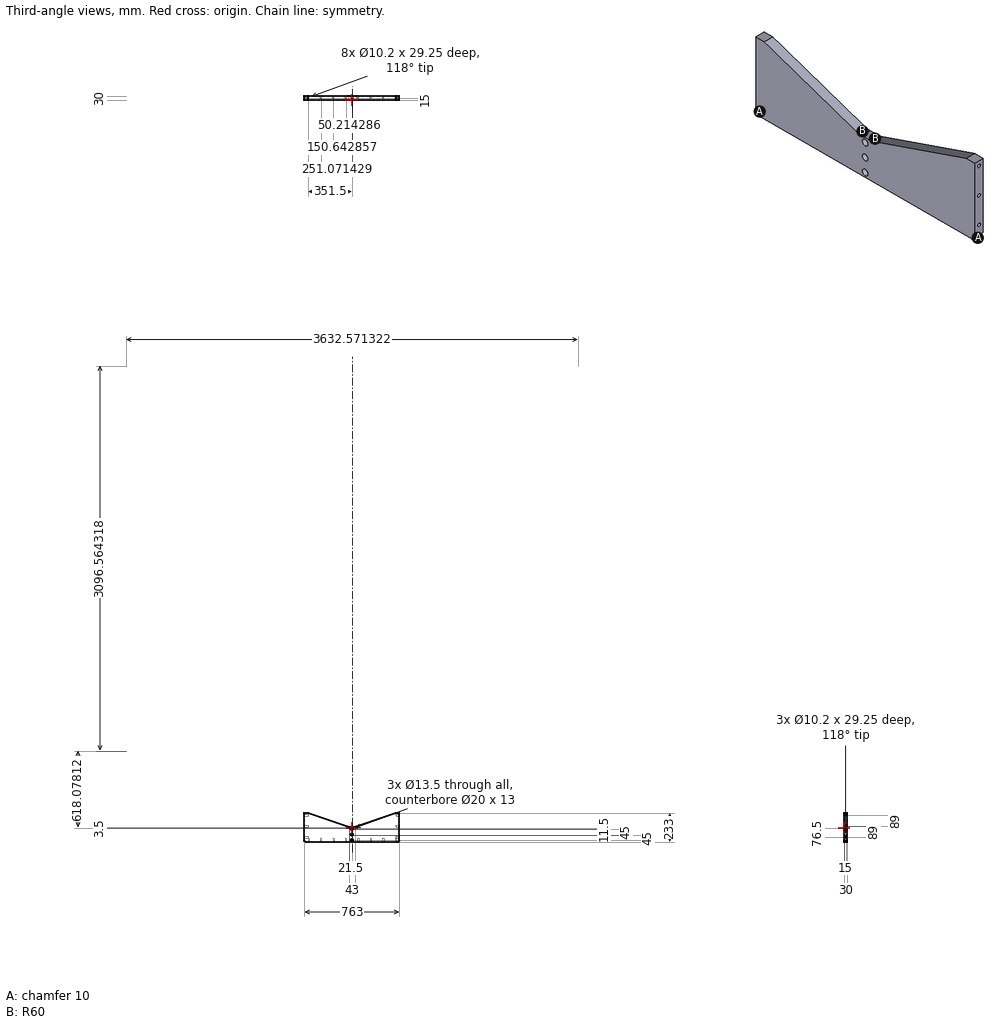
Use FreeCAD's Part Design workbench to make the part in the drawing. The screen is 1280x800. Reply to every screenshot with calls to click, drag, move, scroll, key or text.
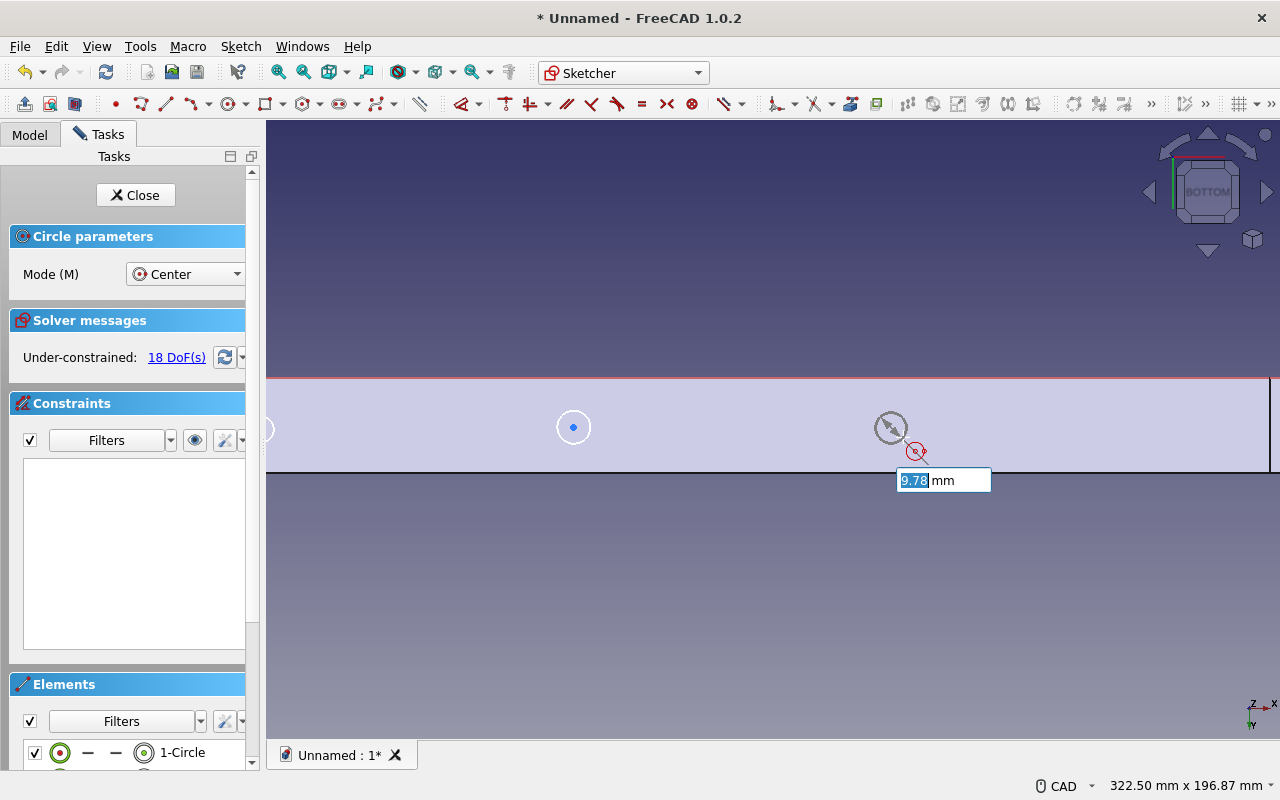
click(902, 437)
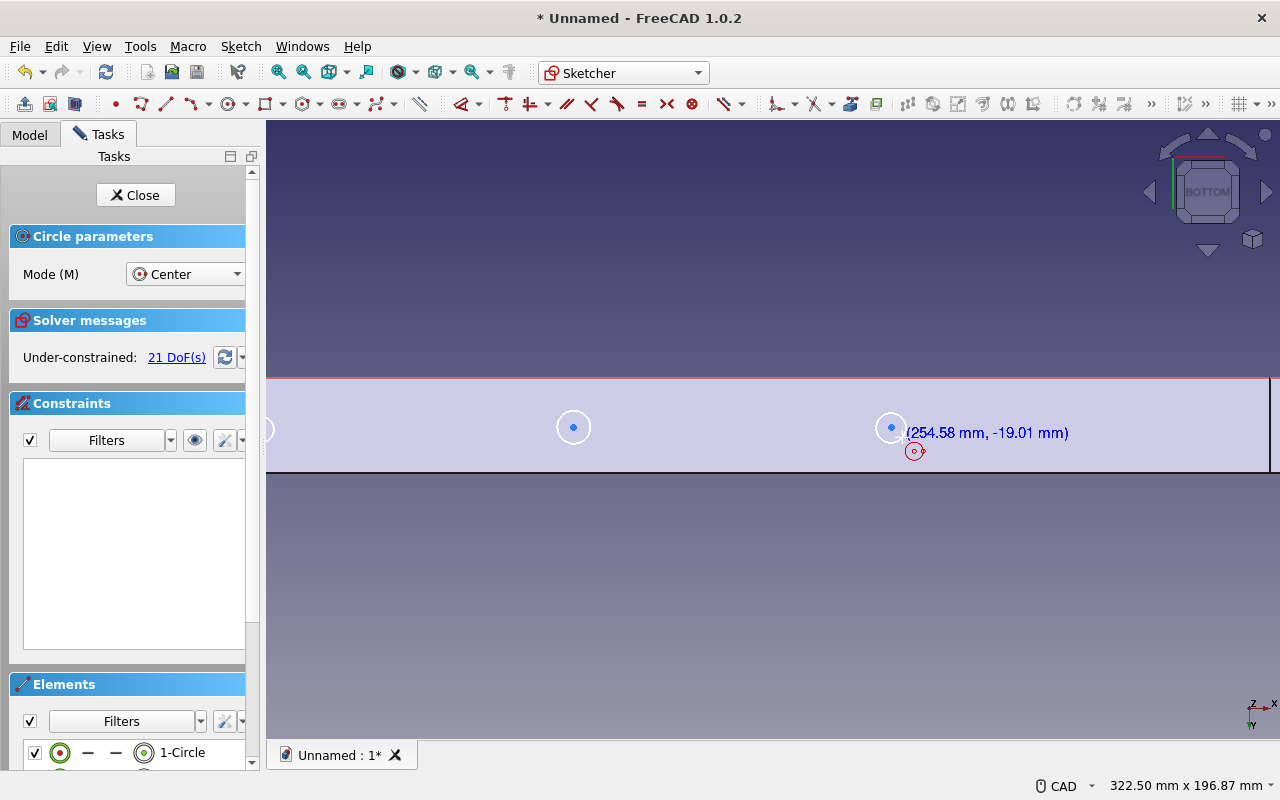
scroll(902, 436, down, 7)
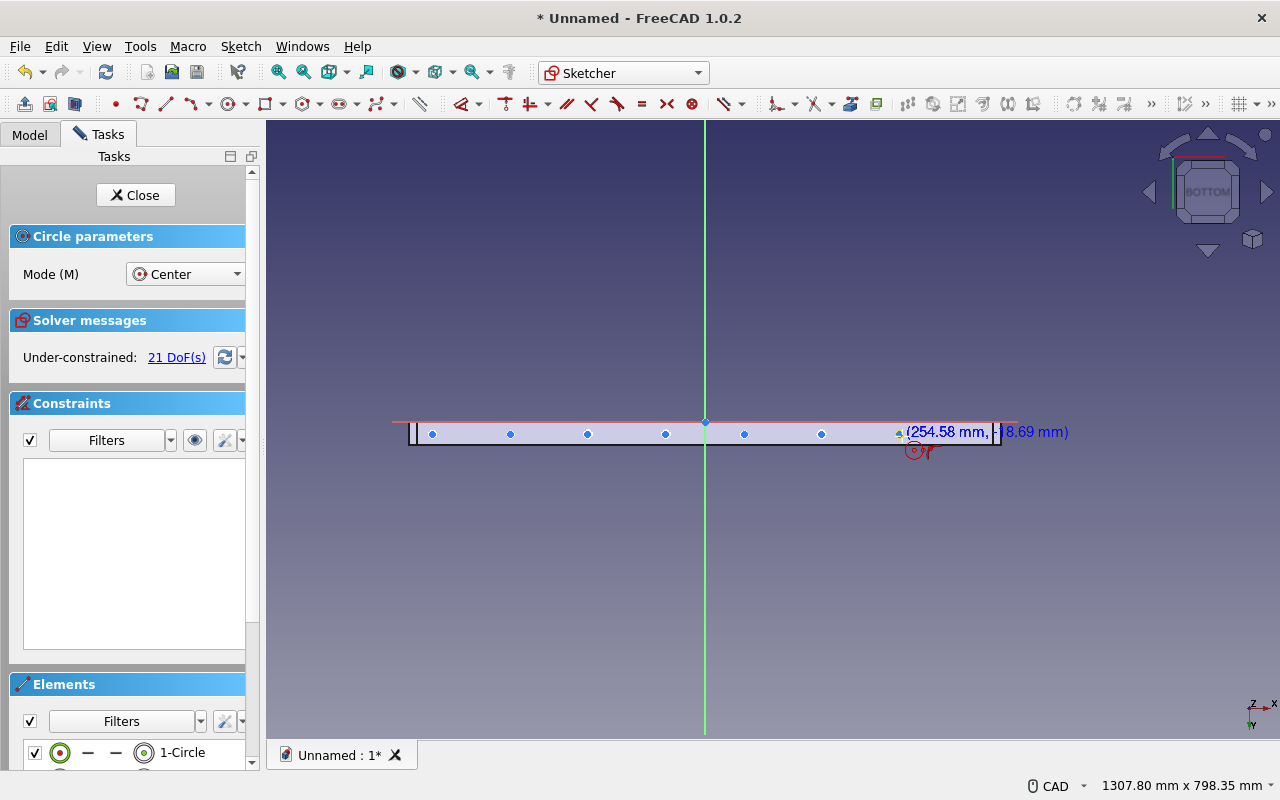
scroll(978, 434, up, 9)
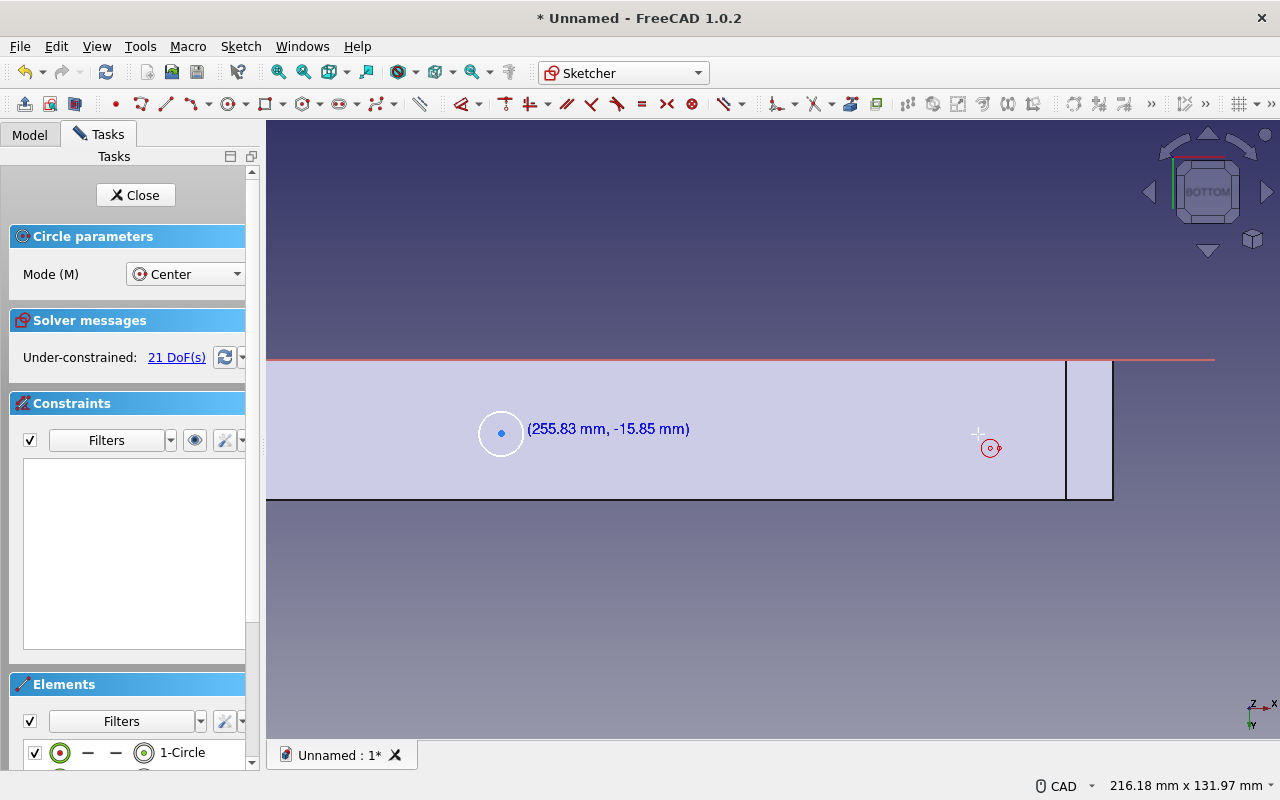
scroll(978, 434, down, 9)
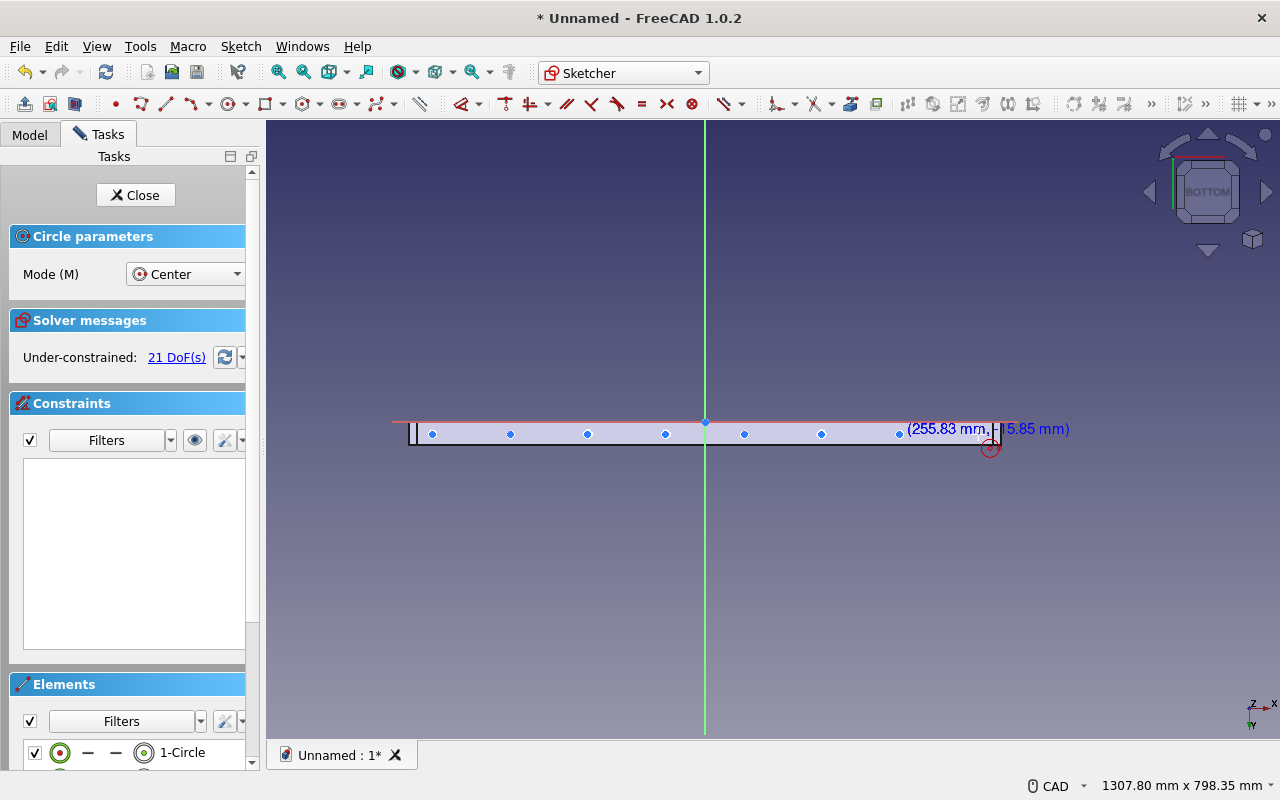
scroll(978, 434, up, 2)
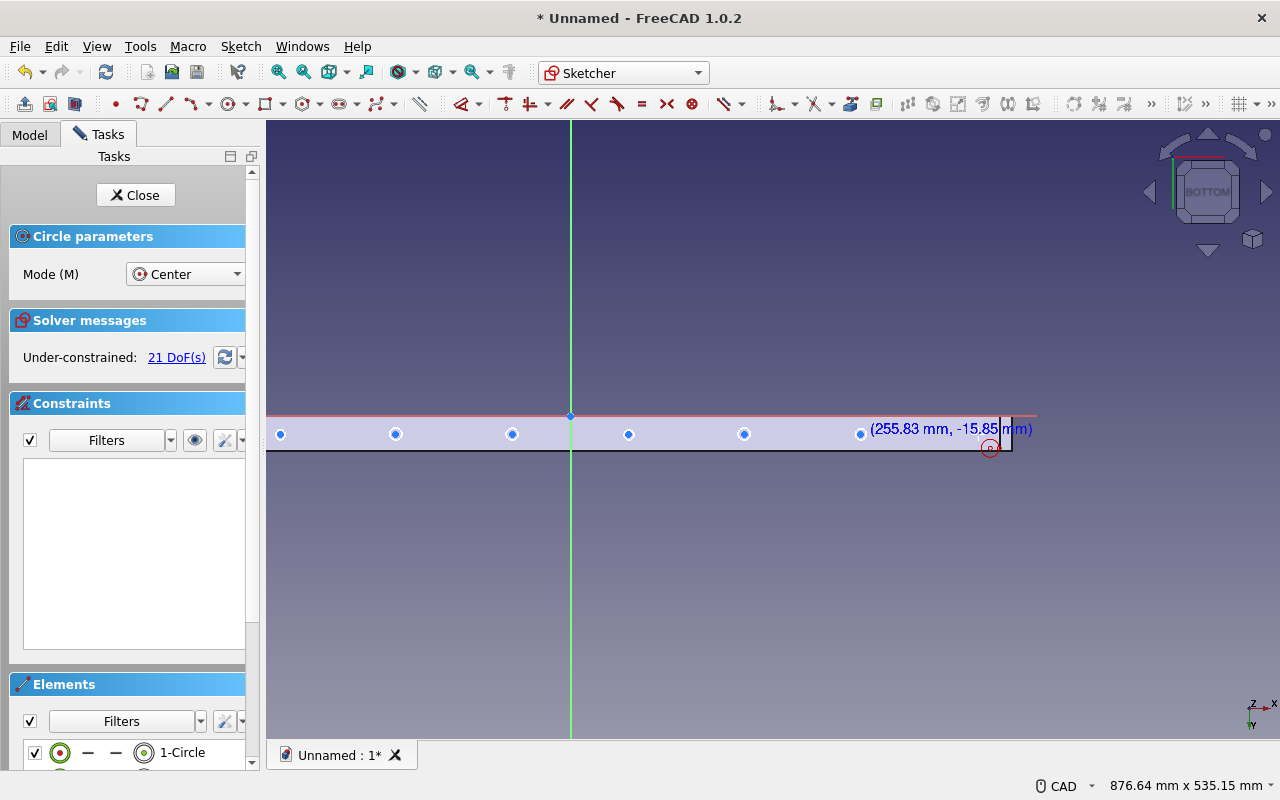
click(977, 433)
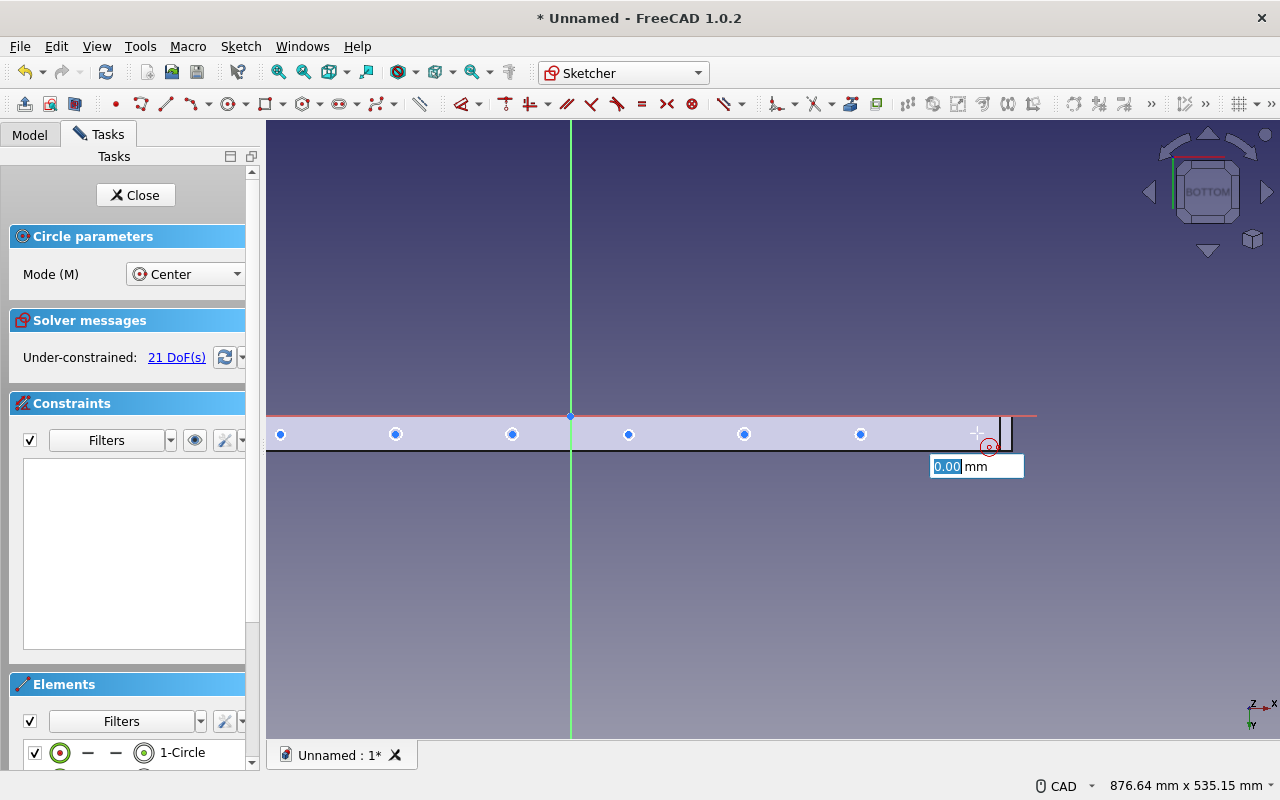
scroll(981, 438, up, 5)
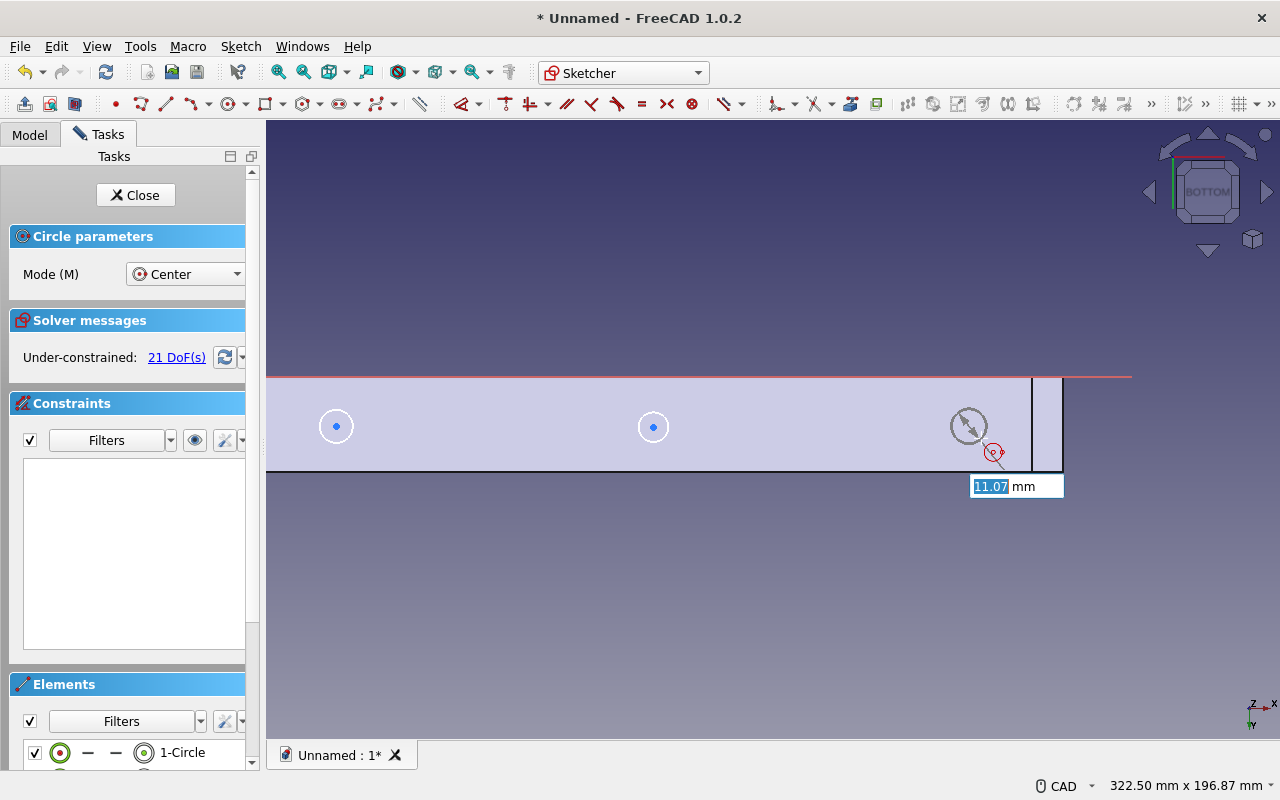
click(980, 436)
key(Escape)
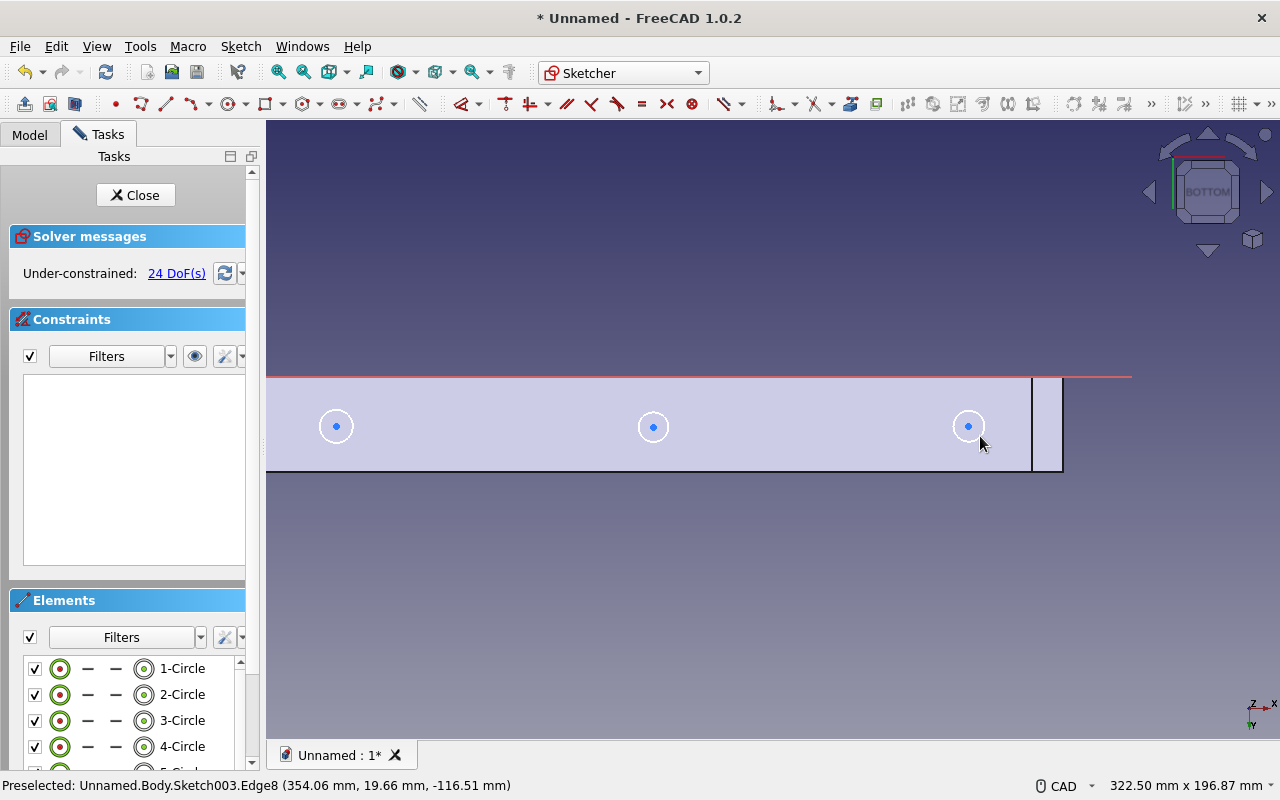
scroll(980, 436, down, 7)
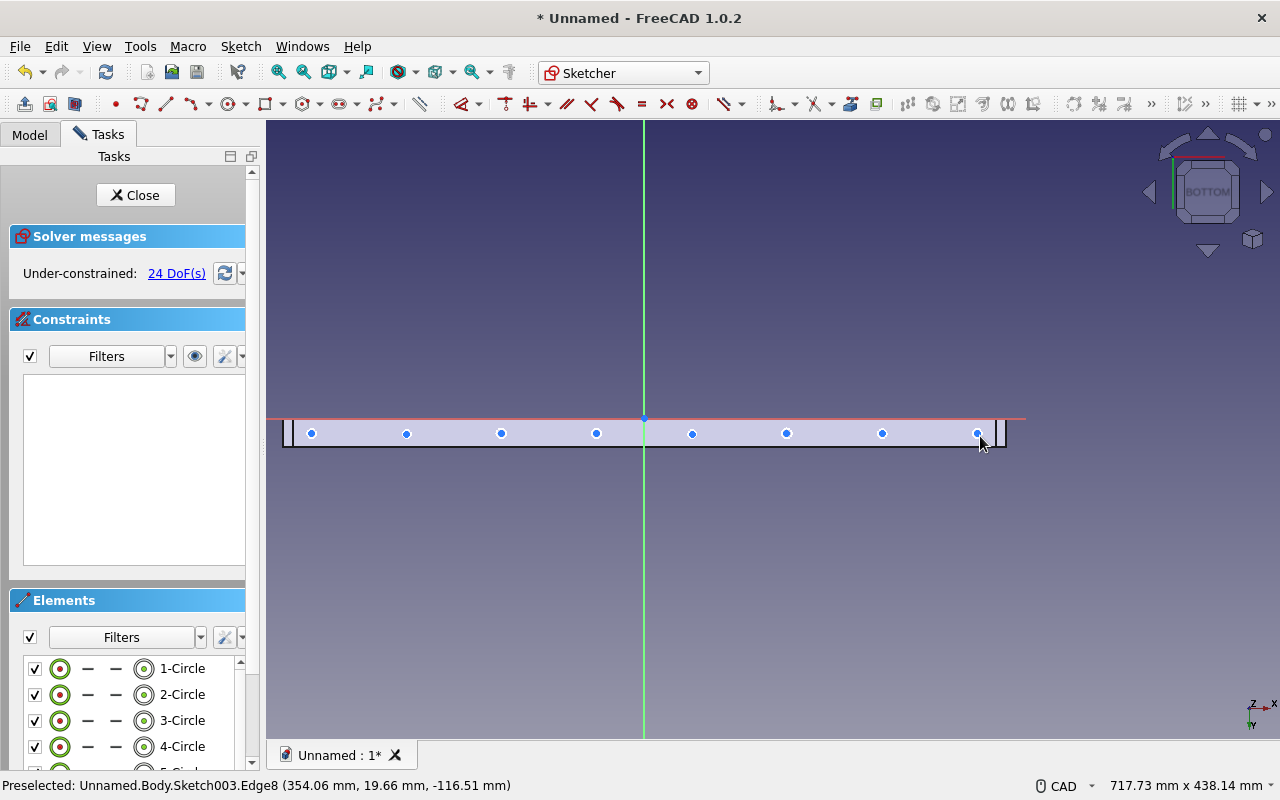
scroll(435, 431, up, 7)